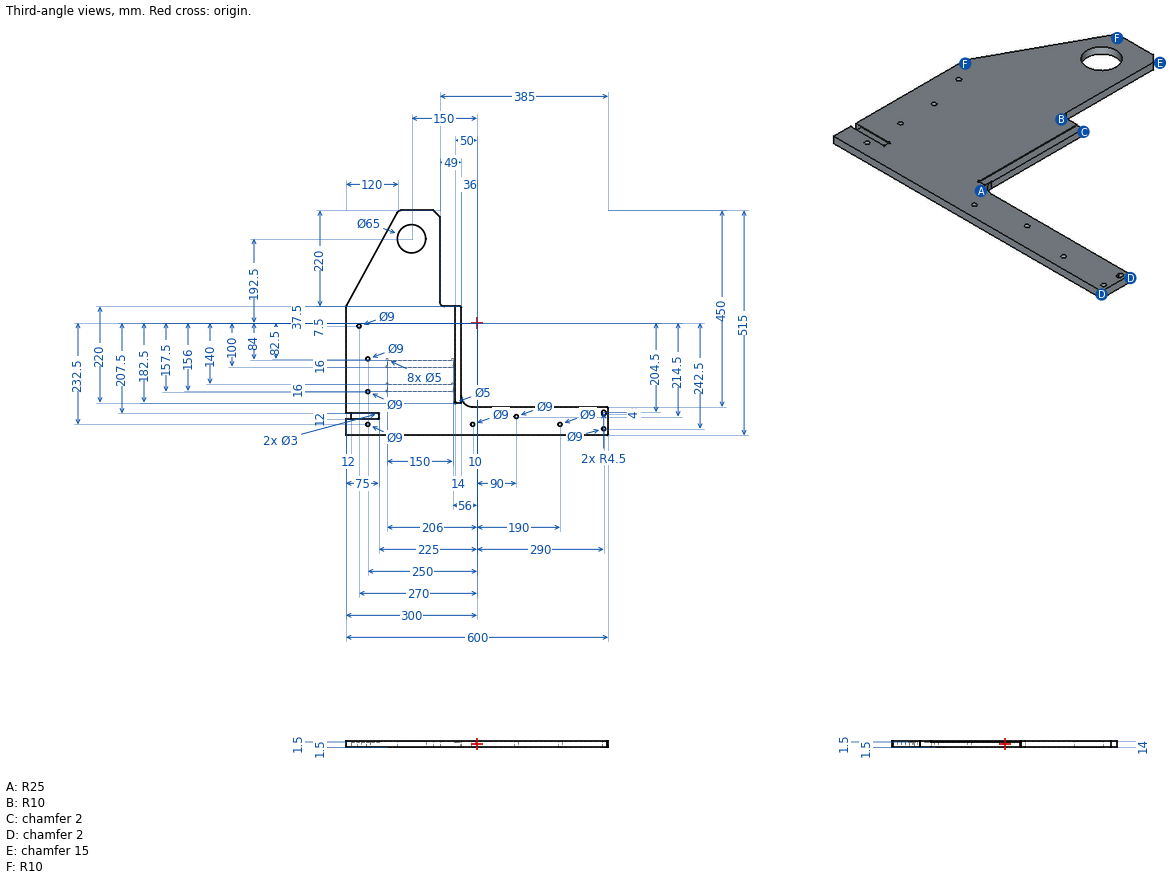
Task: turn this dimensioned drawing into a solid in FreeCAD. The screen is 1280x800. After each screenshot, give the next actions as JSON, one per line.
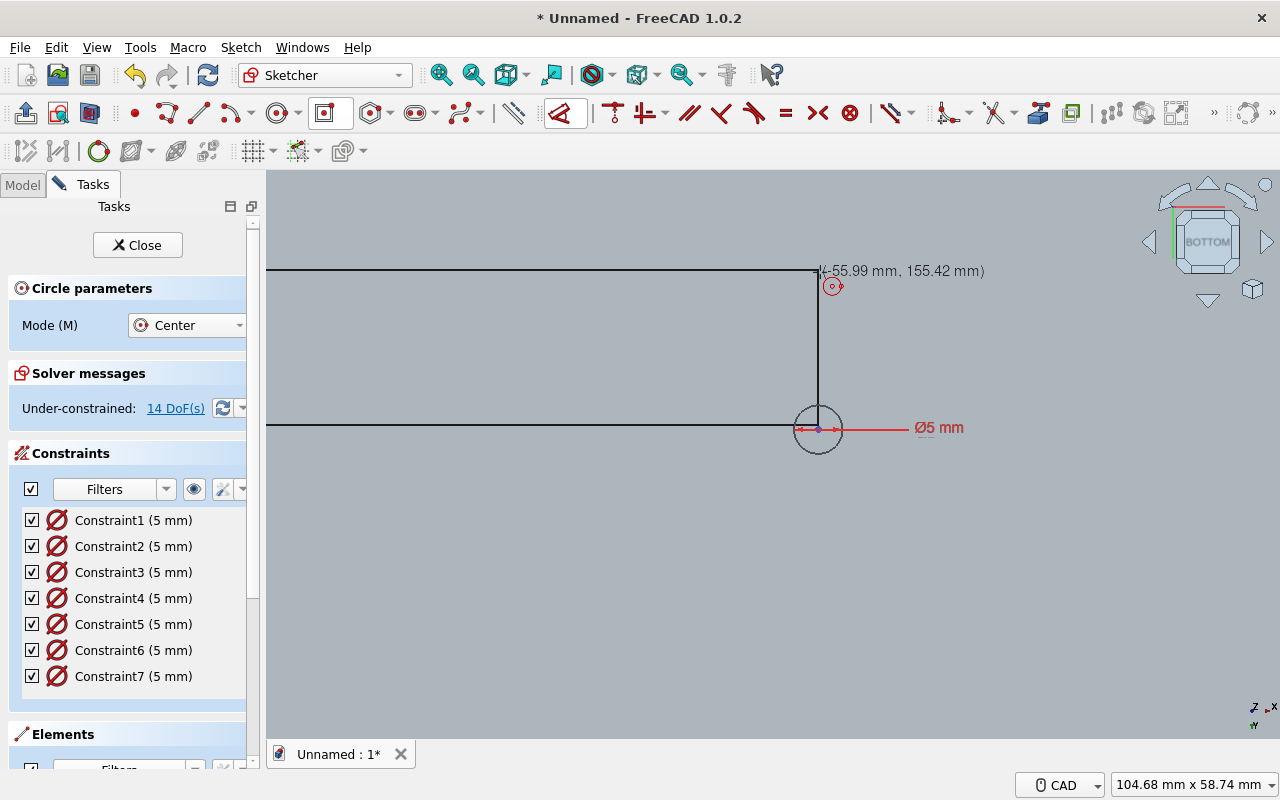
{"action": "scroll", "coordinate": [820, 272], "scroll_direction": "down", "scroll_amount": 7}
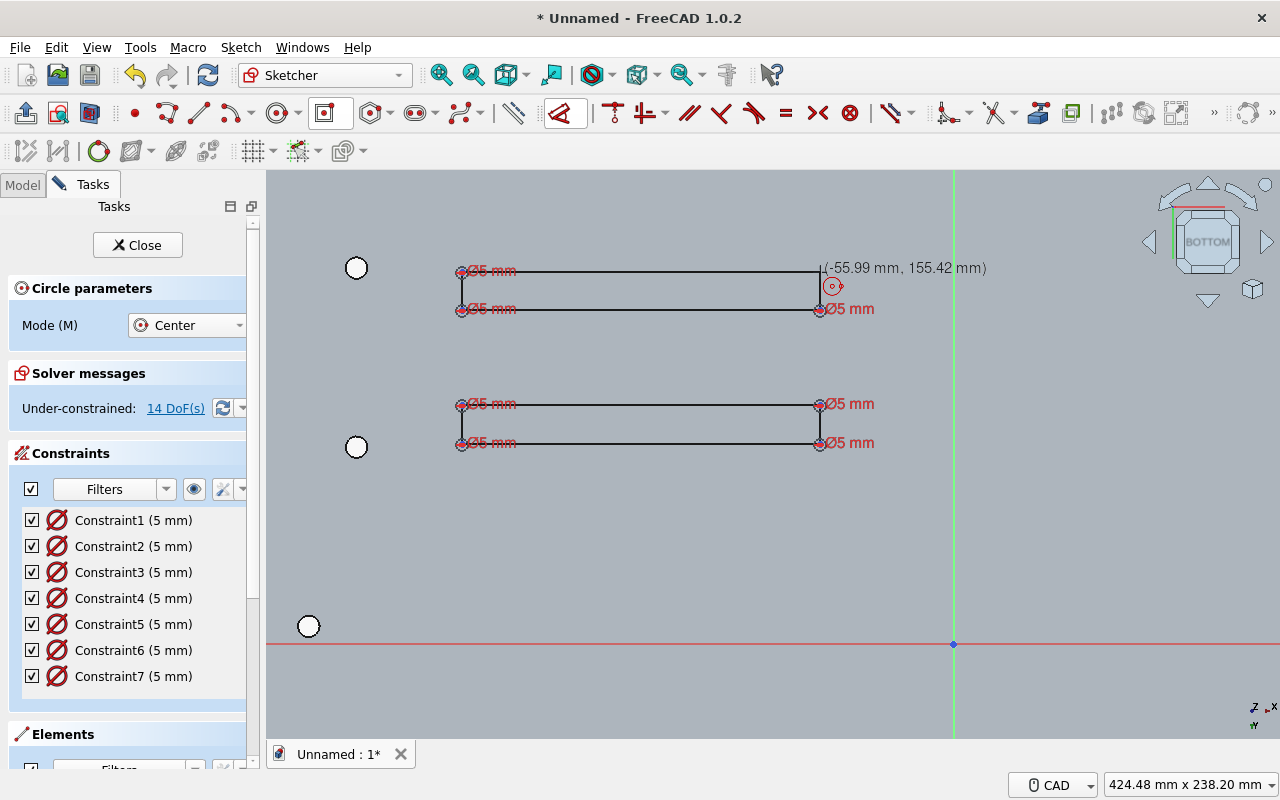
{"action": "left_click", "coordinate": [820, 272]}
{"action": "mouse_move", "coordinate": [824, 267]}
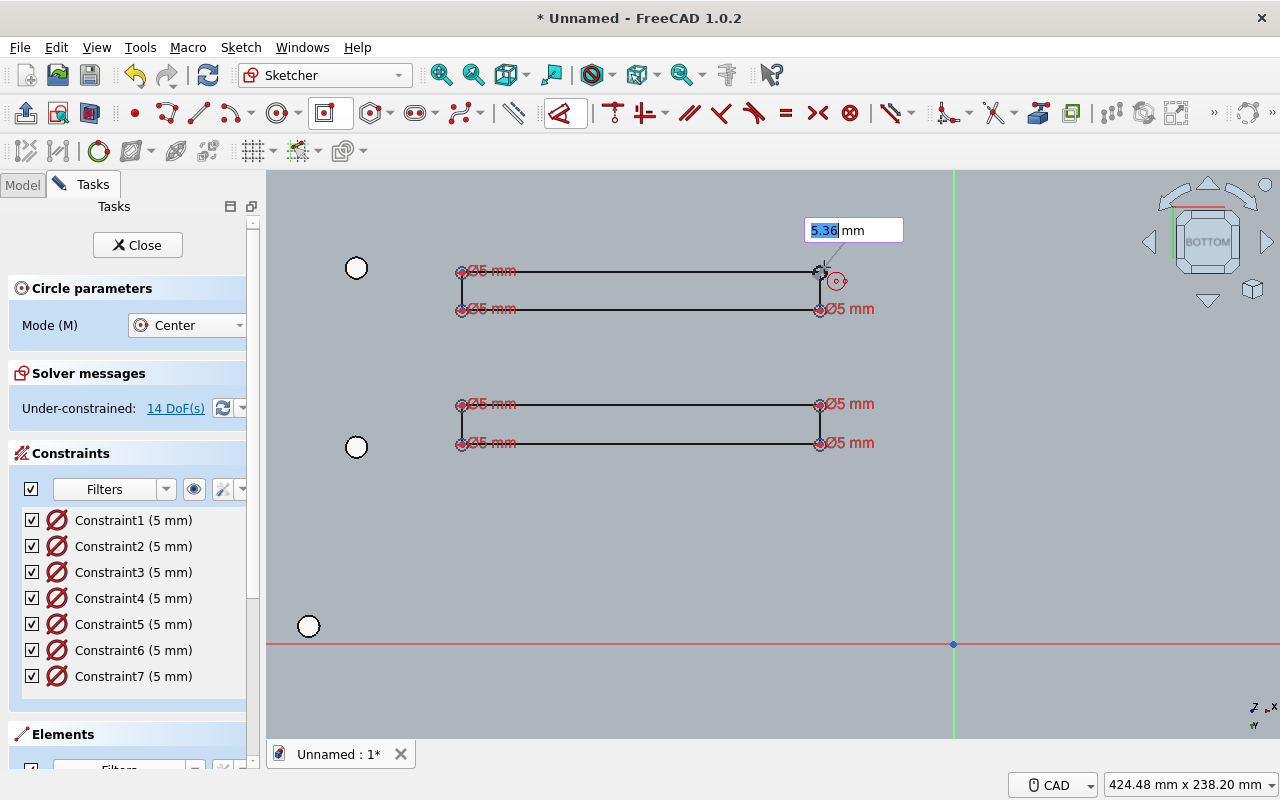
{"action": "type", "text": "5"}
{"action": "key", "text": "Return"}
{"action": "key", "text": "Escape"}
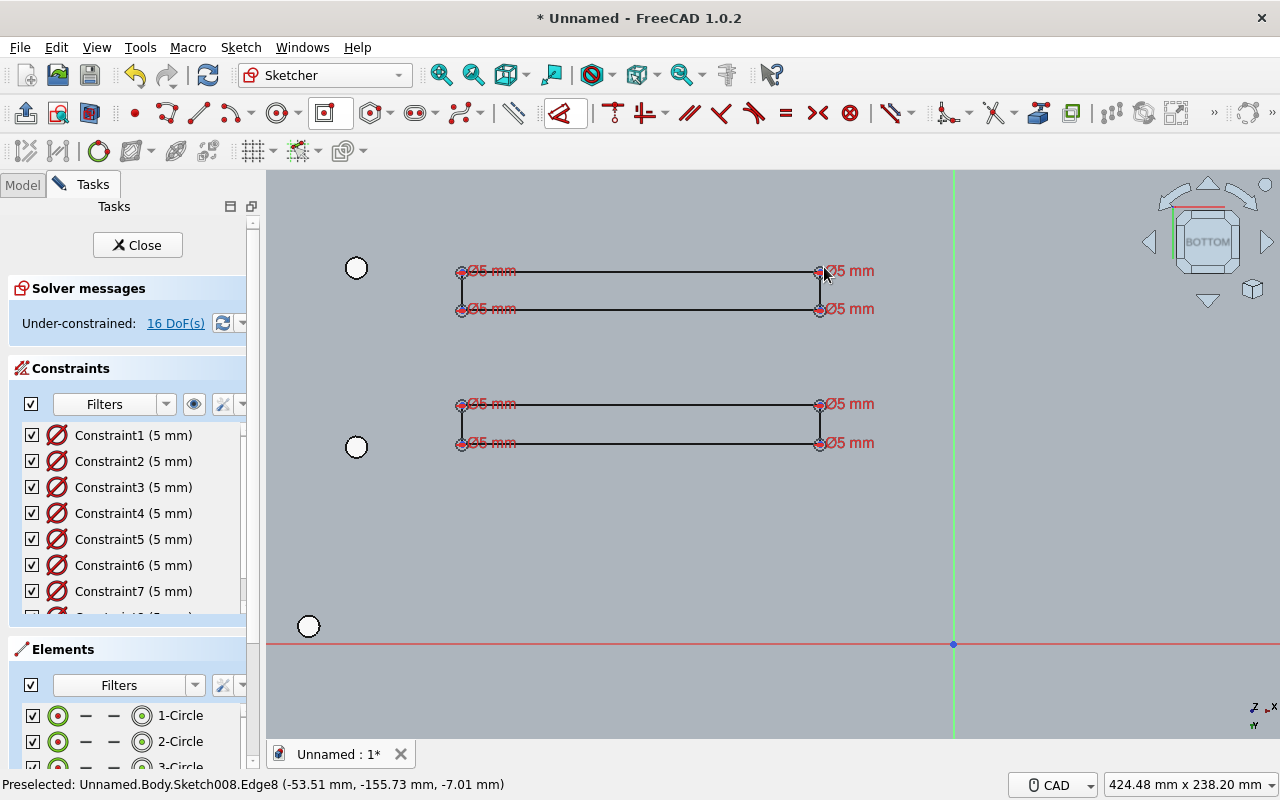
{"action": "left_click", "coordinate": [462, 445]}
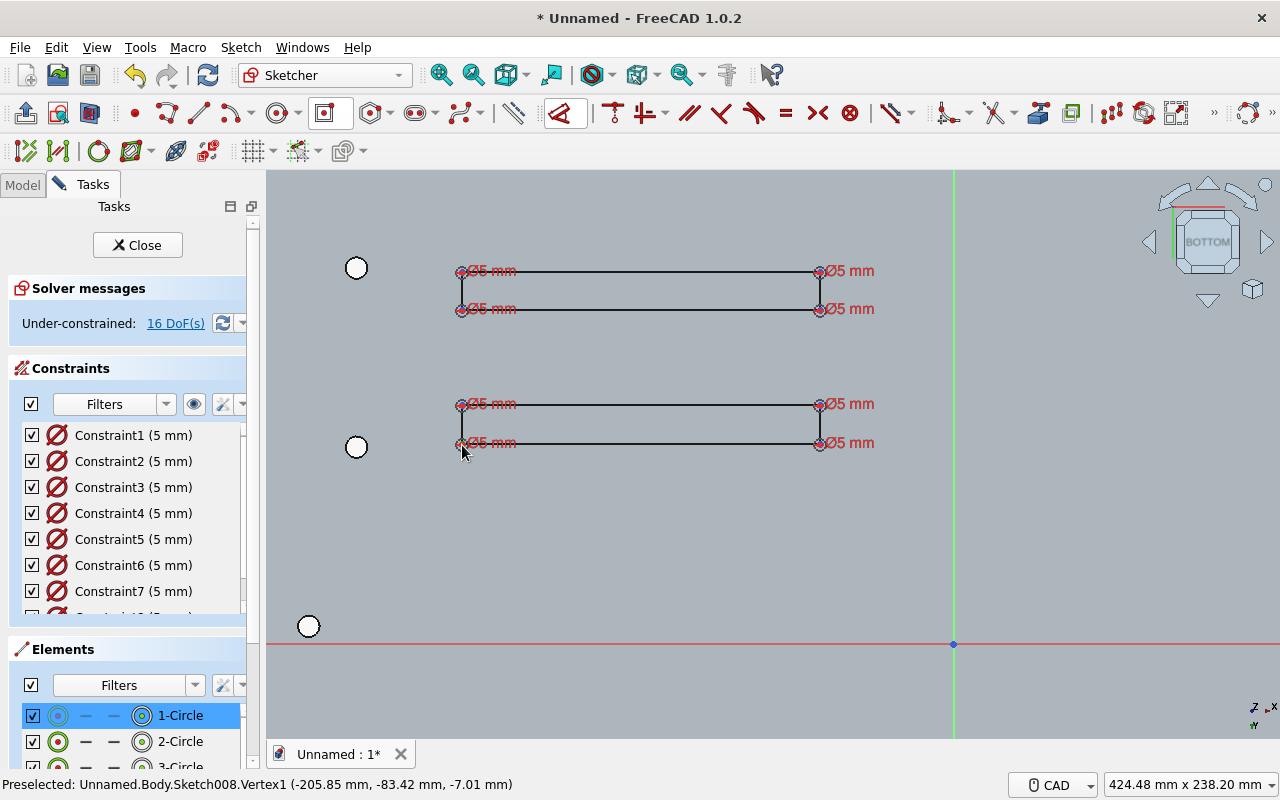
{"action": "left_click", "coordinate": [582, 114]}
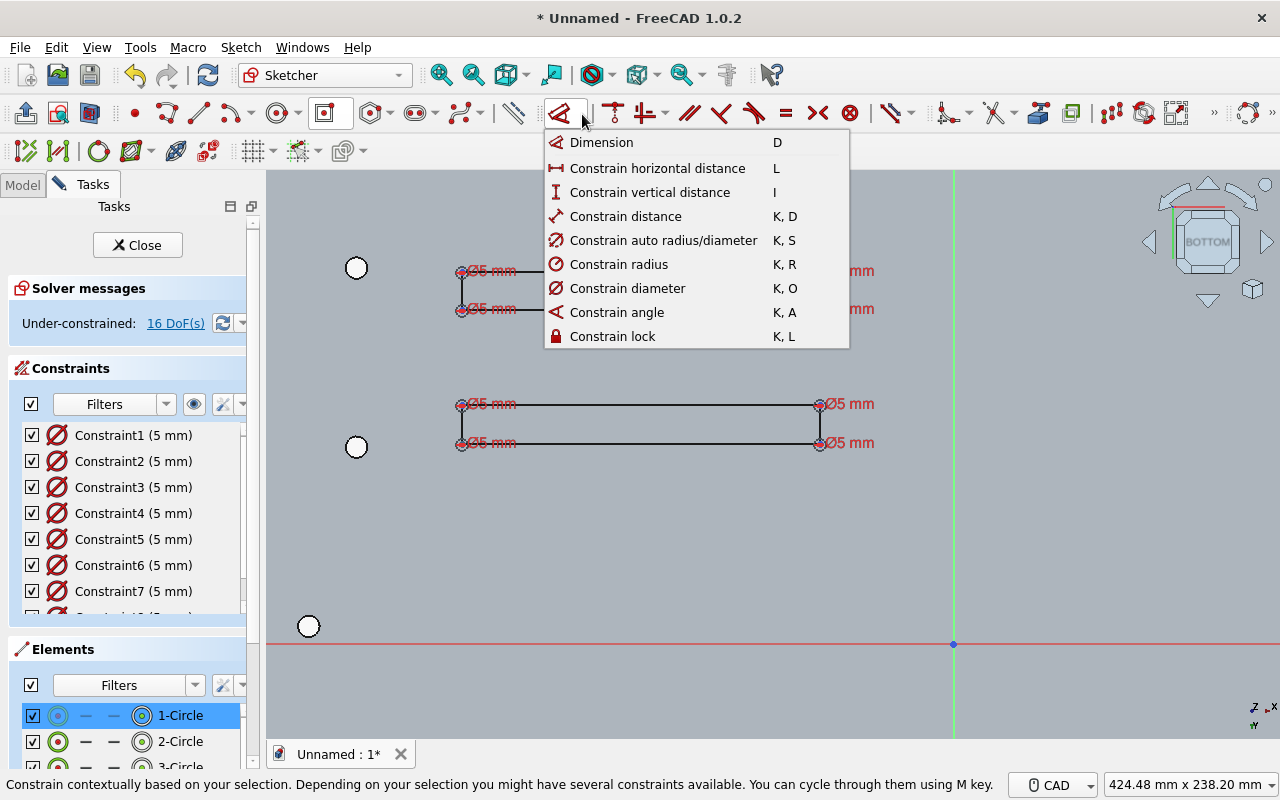
{"action": "left_click", "coordinate": [697, 192]}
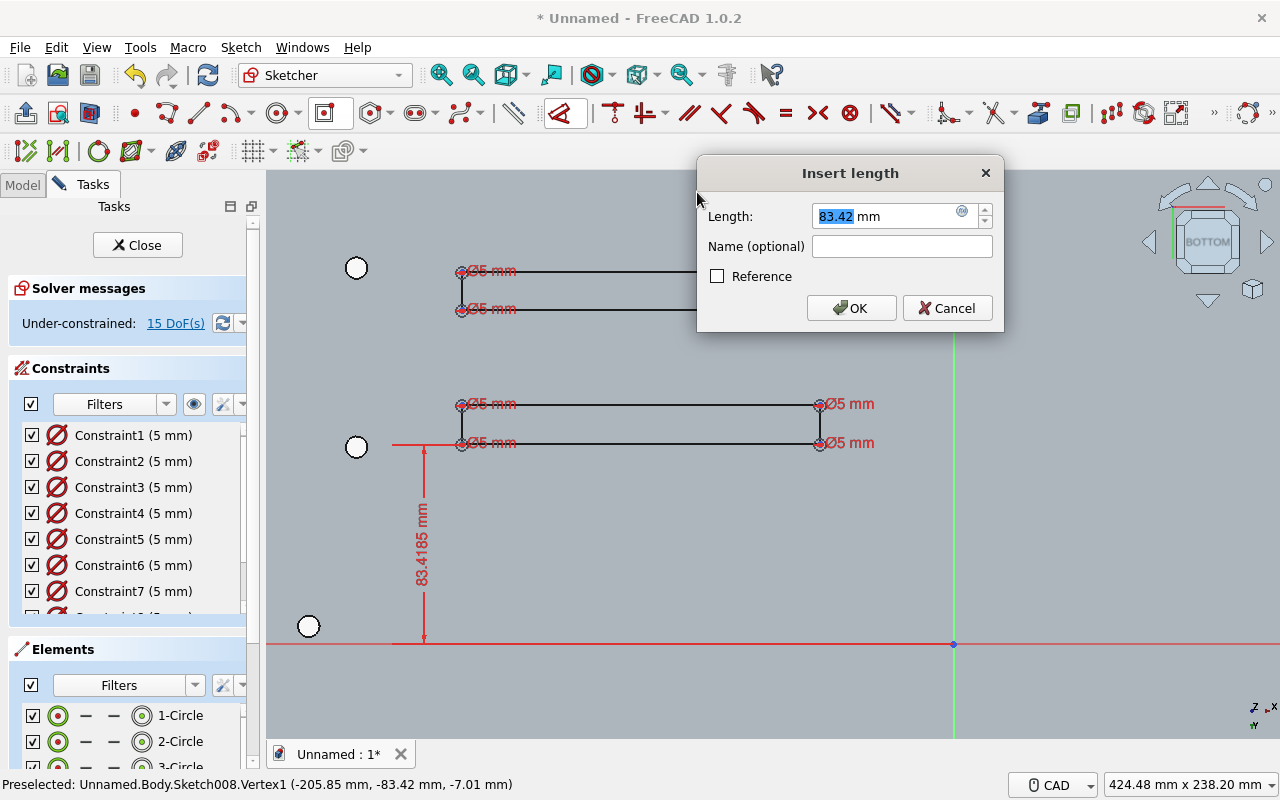
{"action": "type", "text": "84"}
{"action": "key", "text": "Return"}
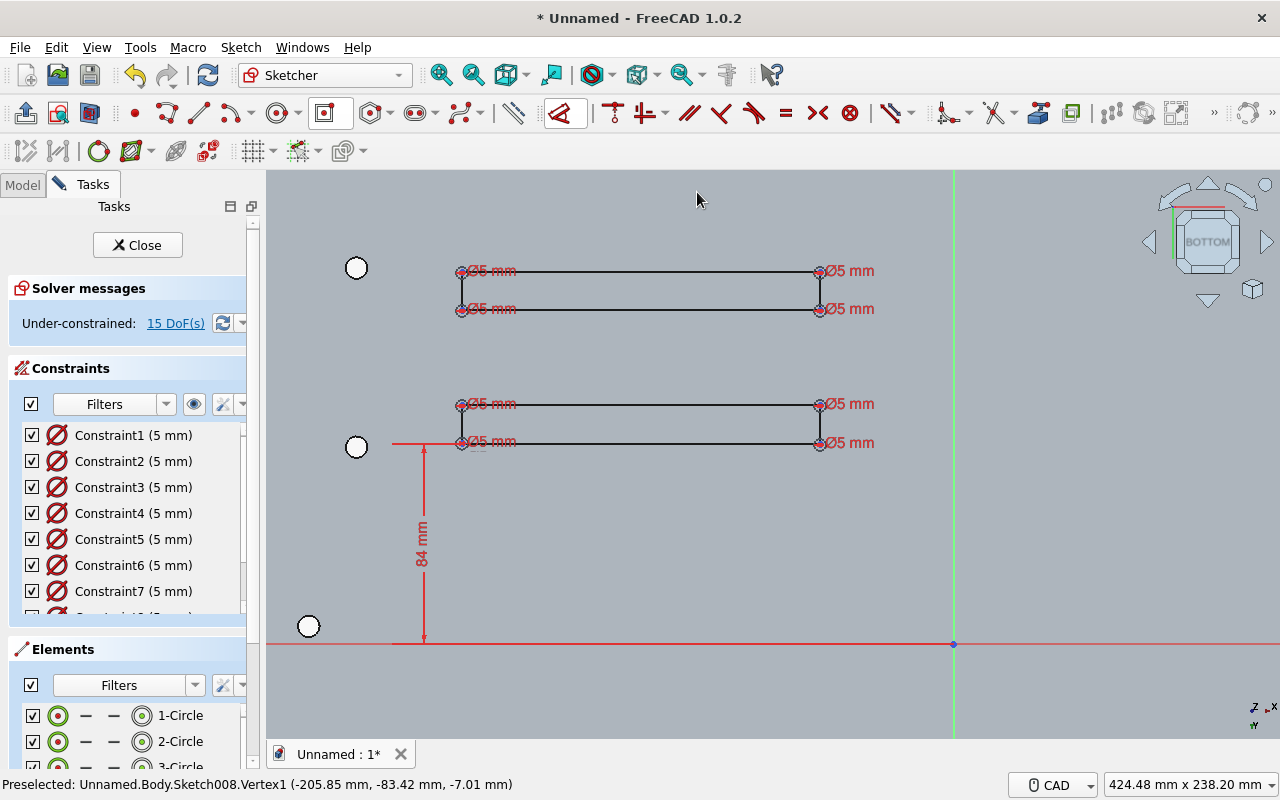
{"action": "left_click", "coordinate": [820, 445]}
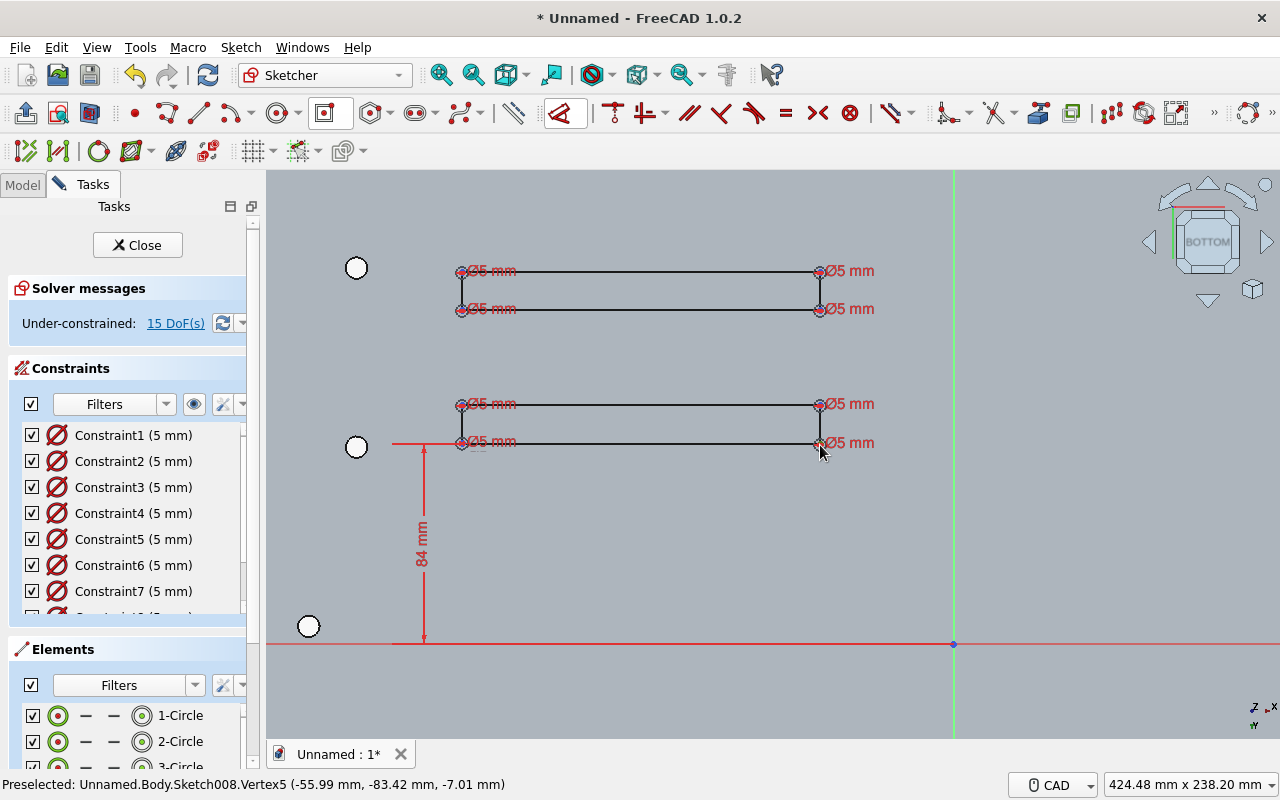
{"action": "left_click", "coordinate": [582, 114]}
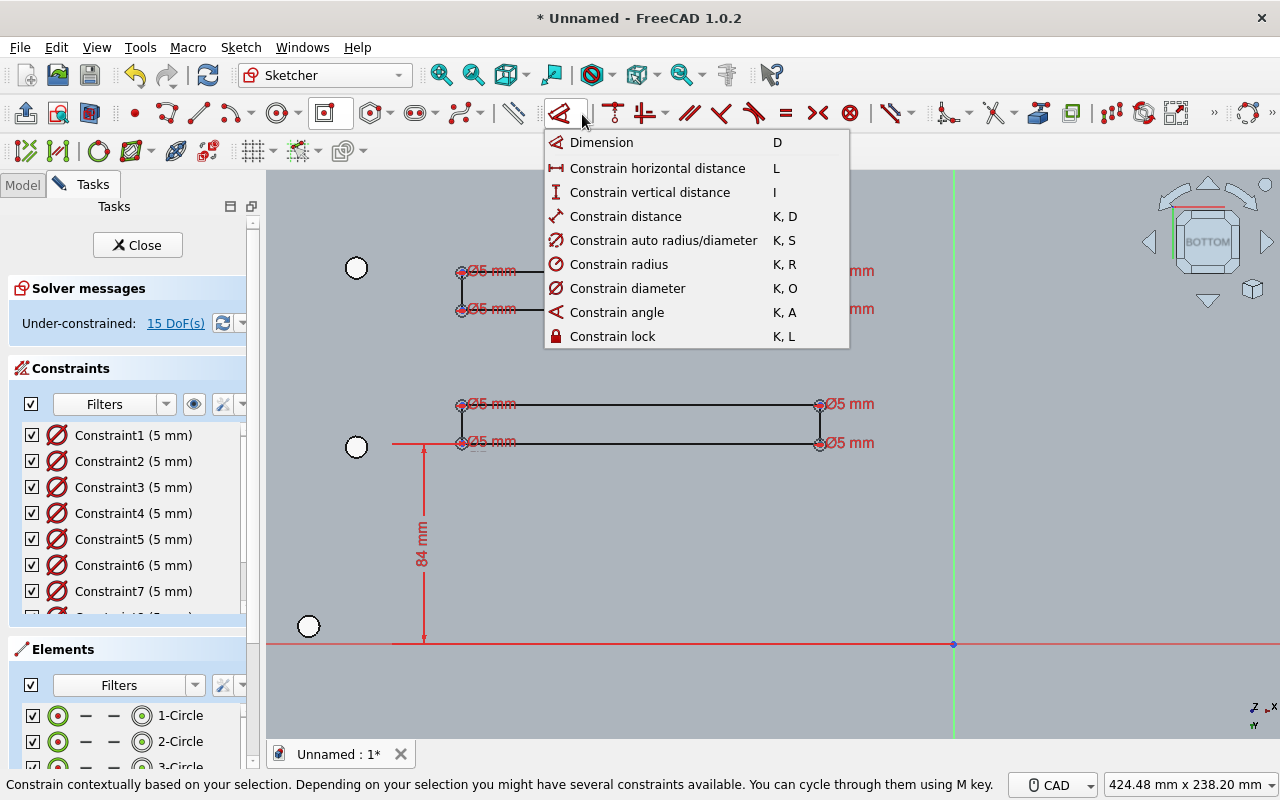
{"action": "left_click", "coordinate": [697, 168]}